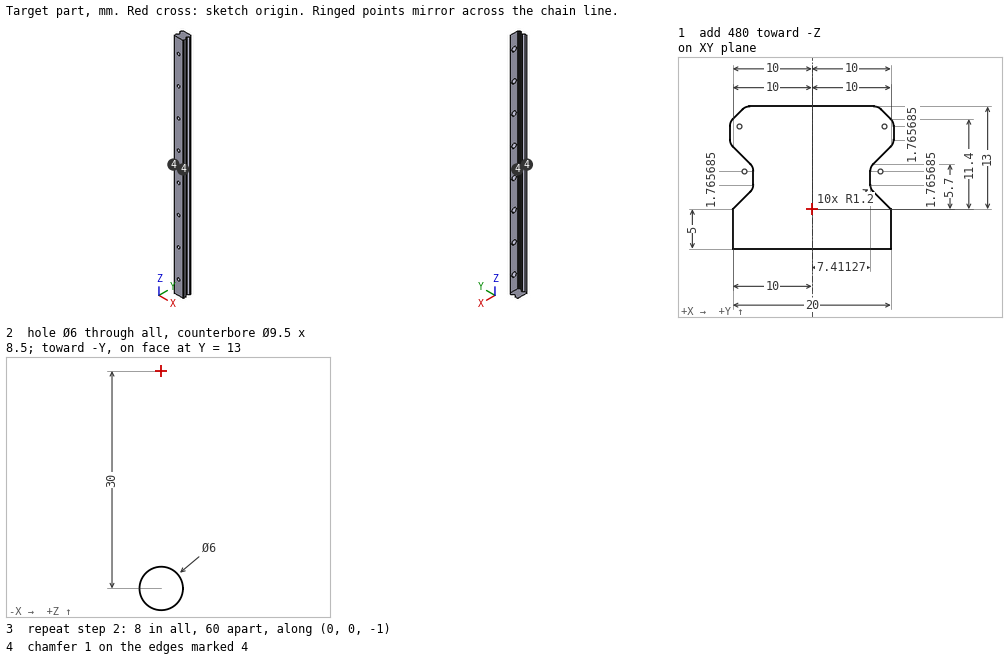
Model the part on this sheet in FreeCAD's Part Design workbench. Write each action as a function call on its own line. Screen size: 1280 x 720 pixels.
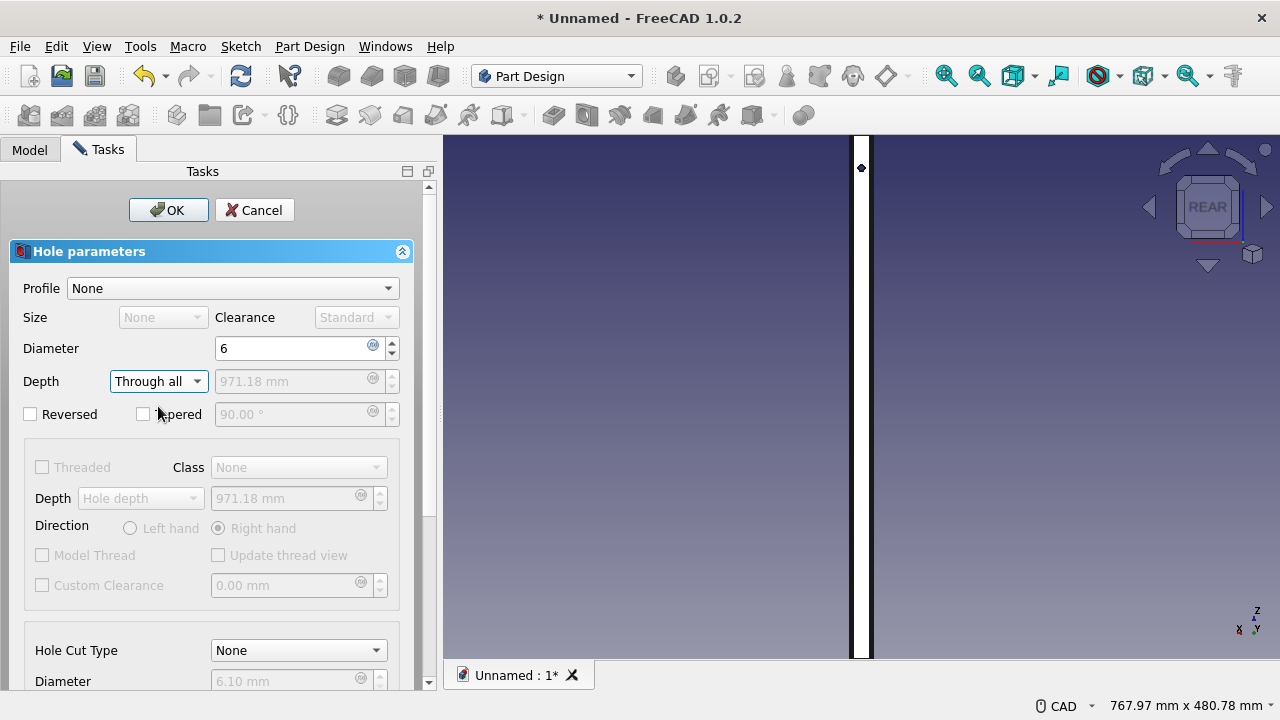
click(300, 650)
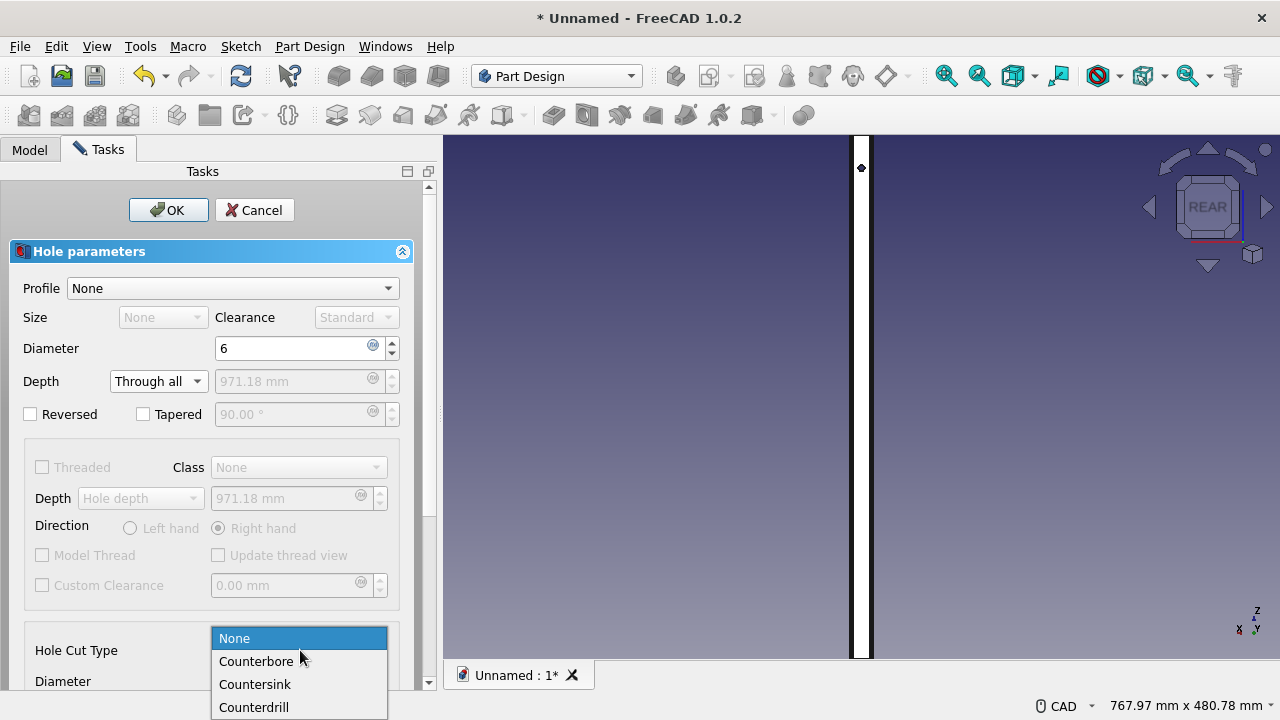
click(298, 662)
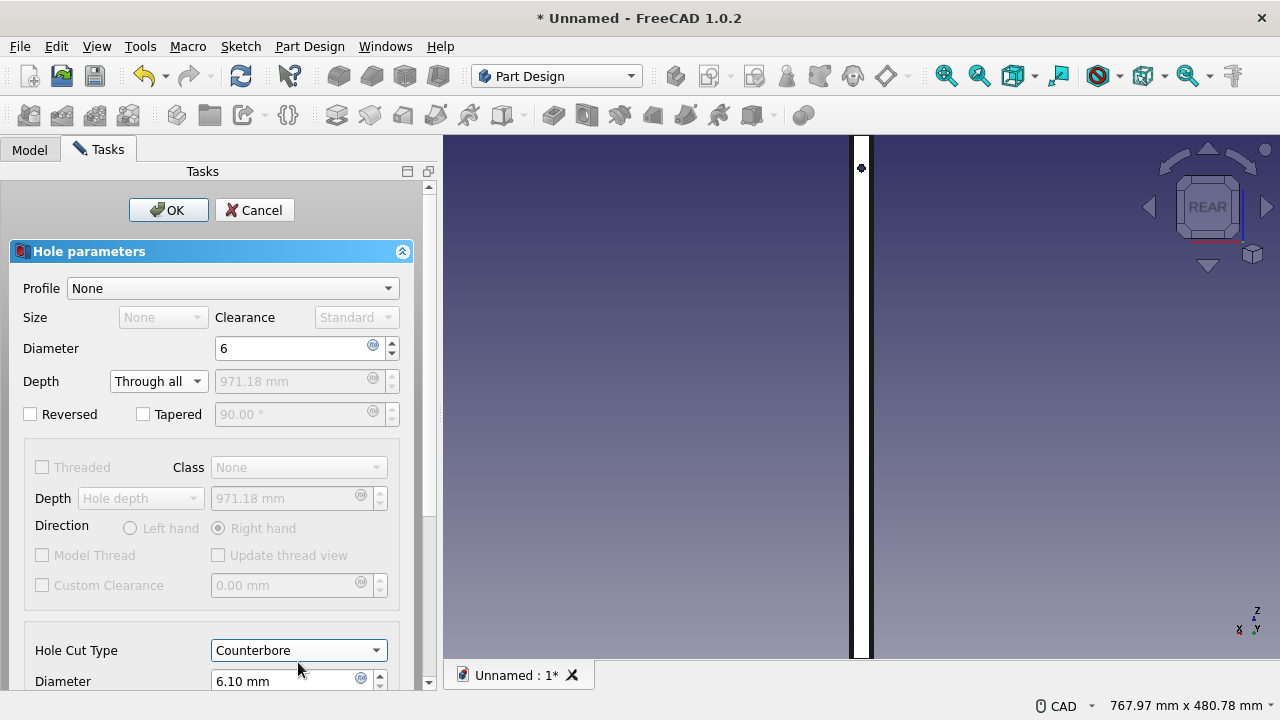
scroll(429, 436, down, 2)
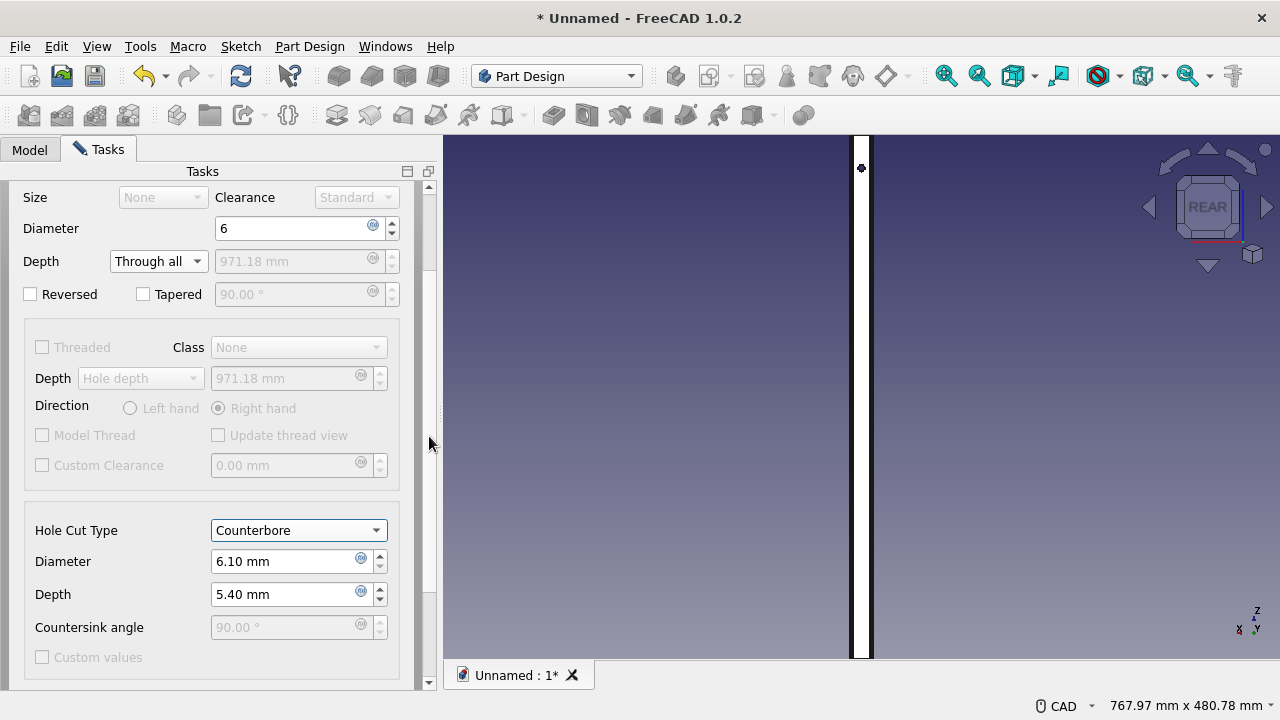
triple_click(292, 562)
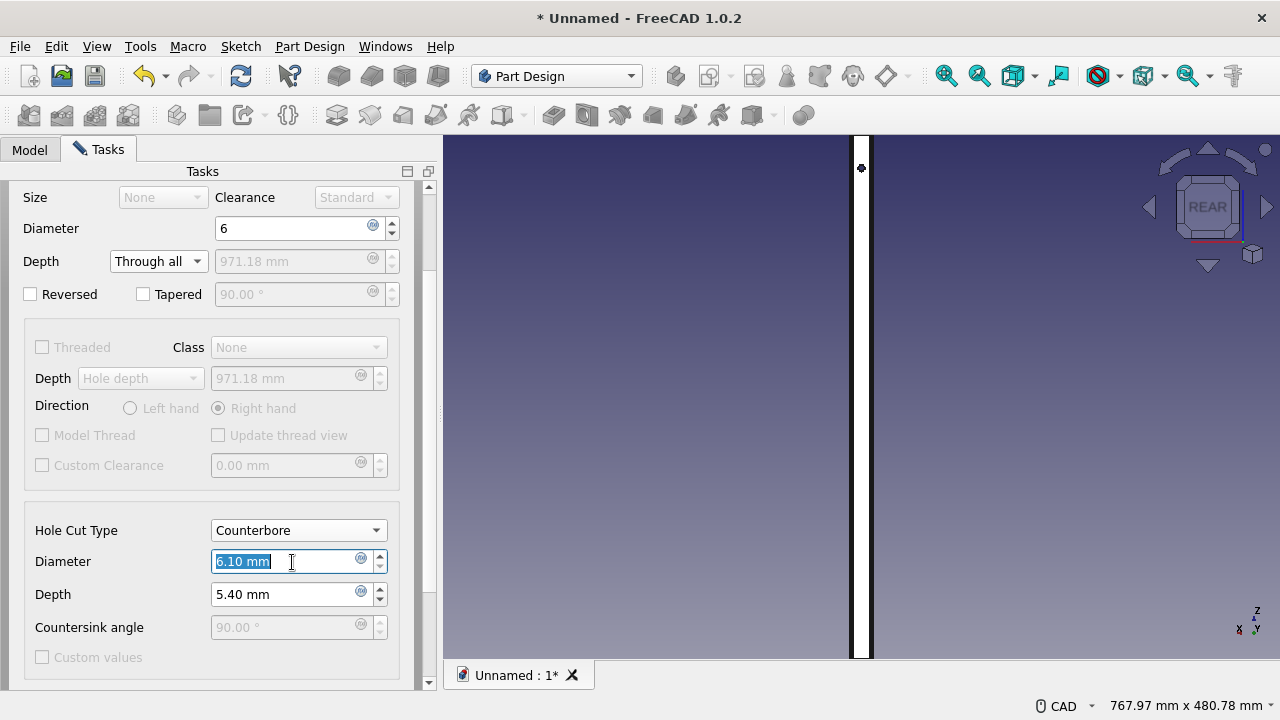
text(9.5)
key(Tab)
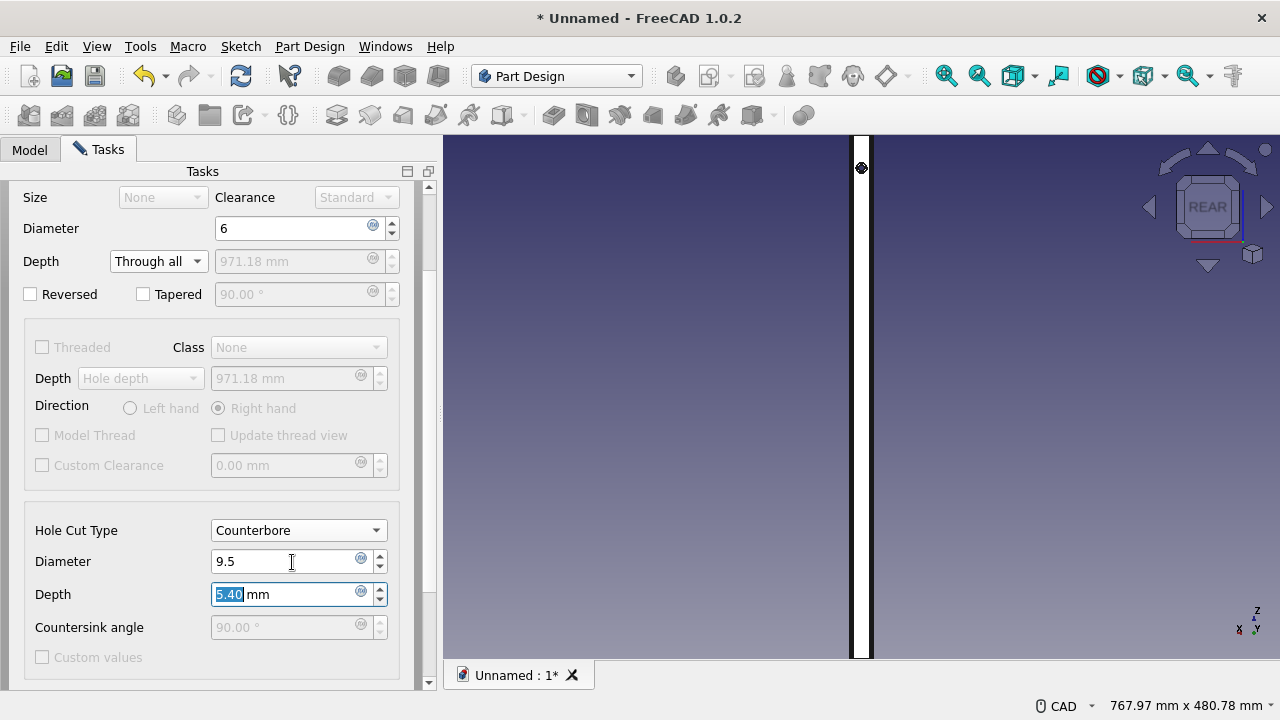
text(8.5)
key(Tab)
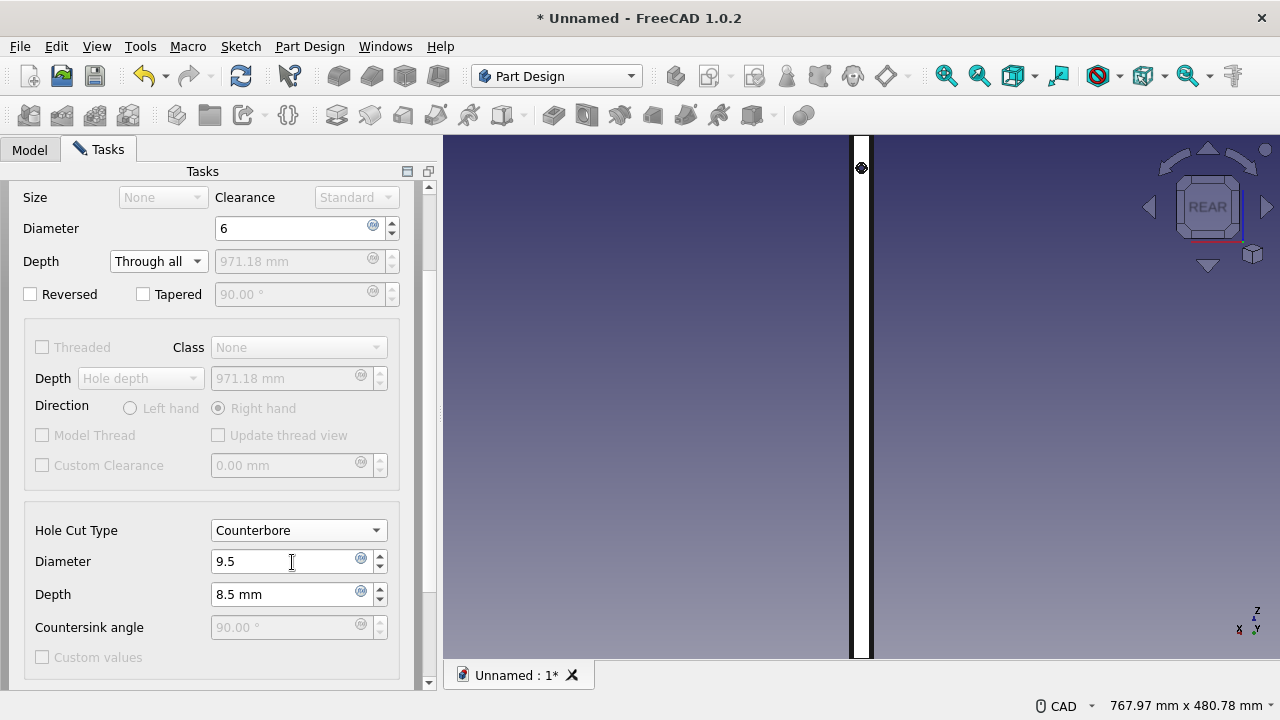
scroll(429, 436, up, 3)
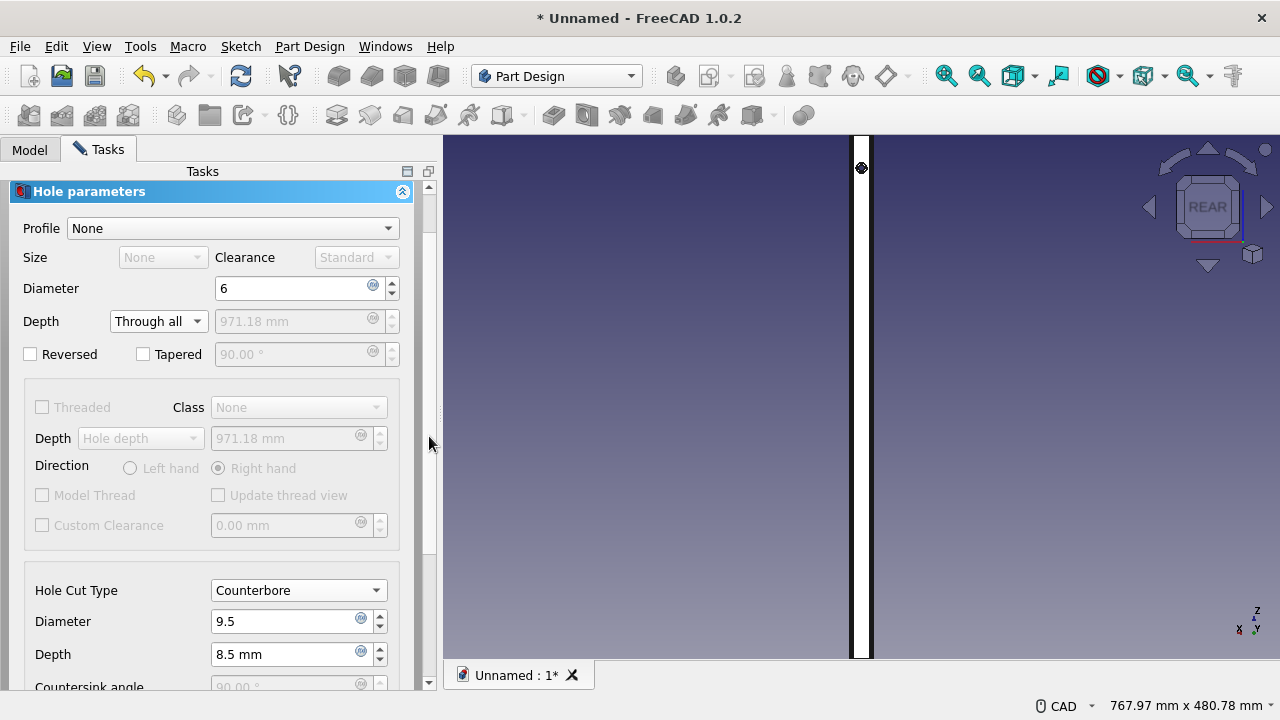
click(169, 210)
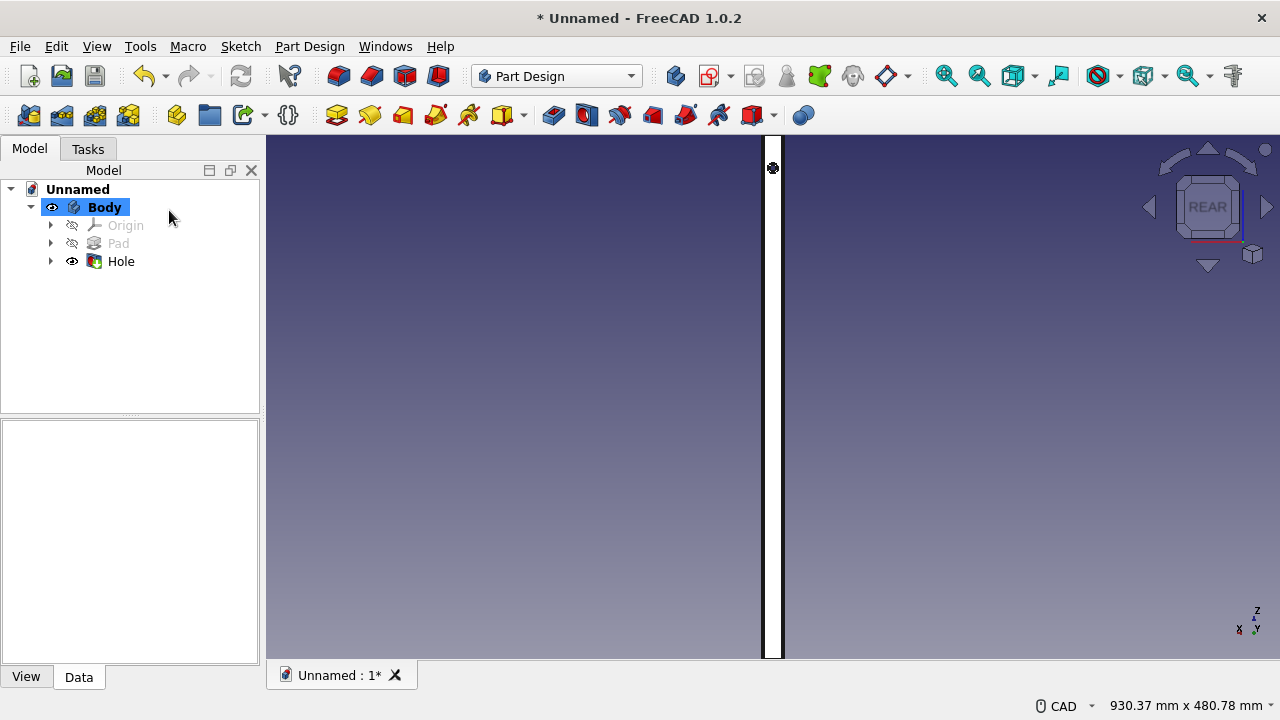
key(v)
key(f)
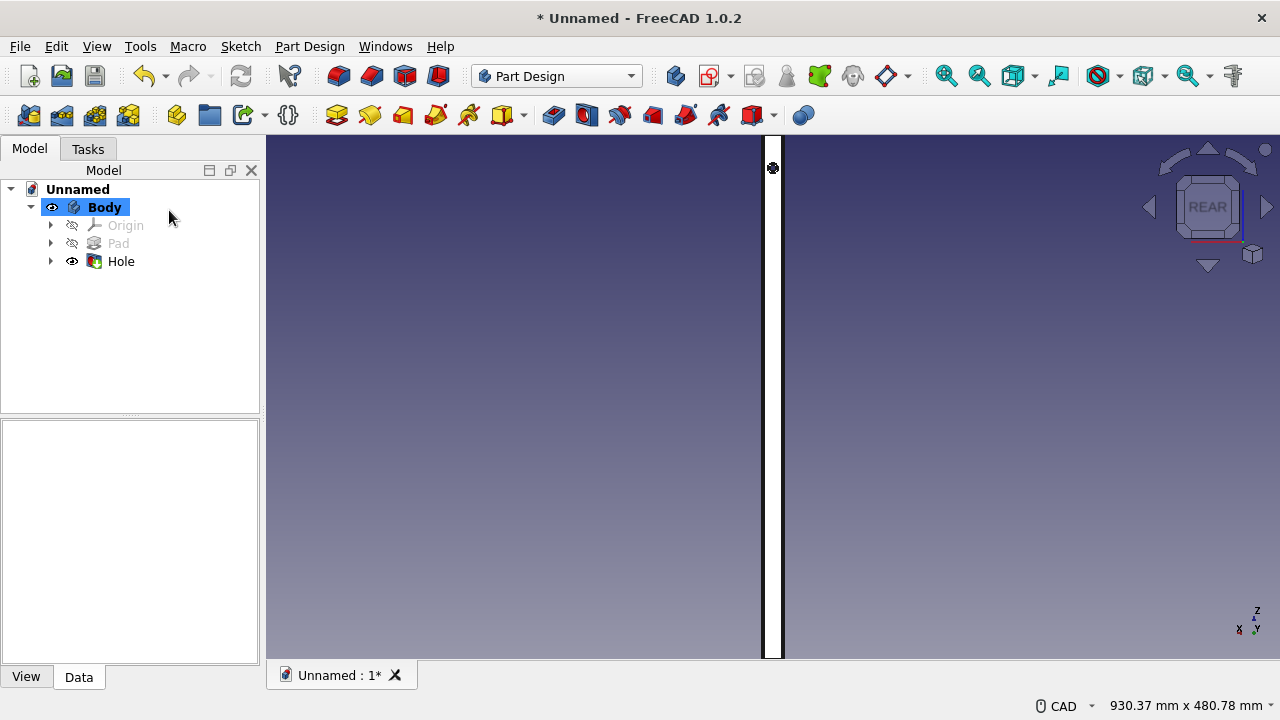
click(117, 261)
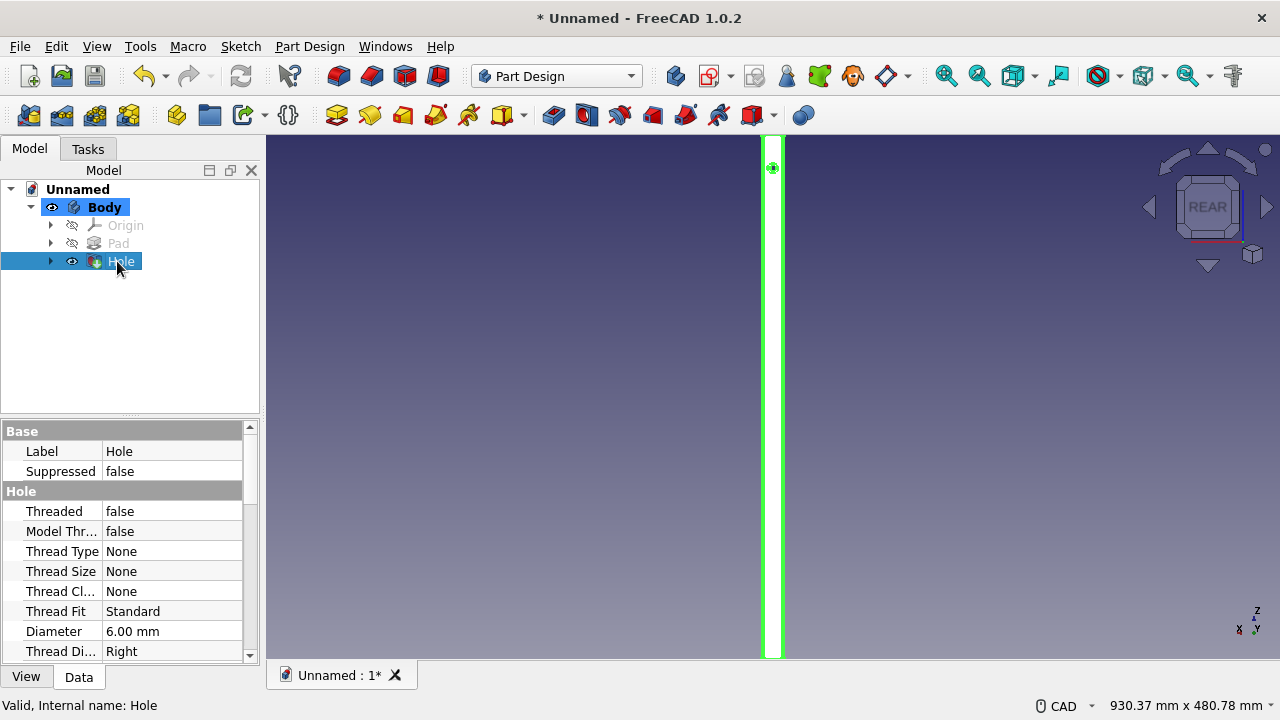
click(62, 116)